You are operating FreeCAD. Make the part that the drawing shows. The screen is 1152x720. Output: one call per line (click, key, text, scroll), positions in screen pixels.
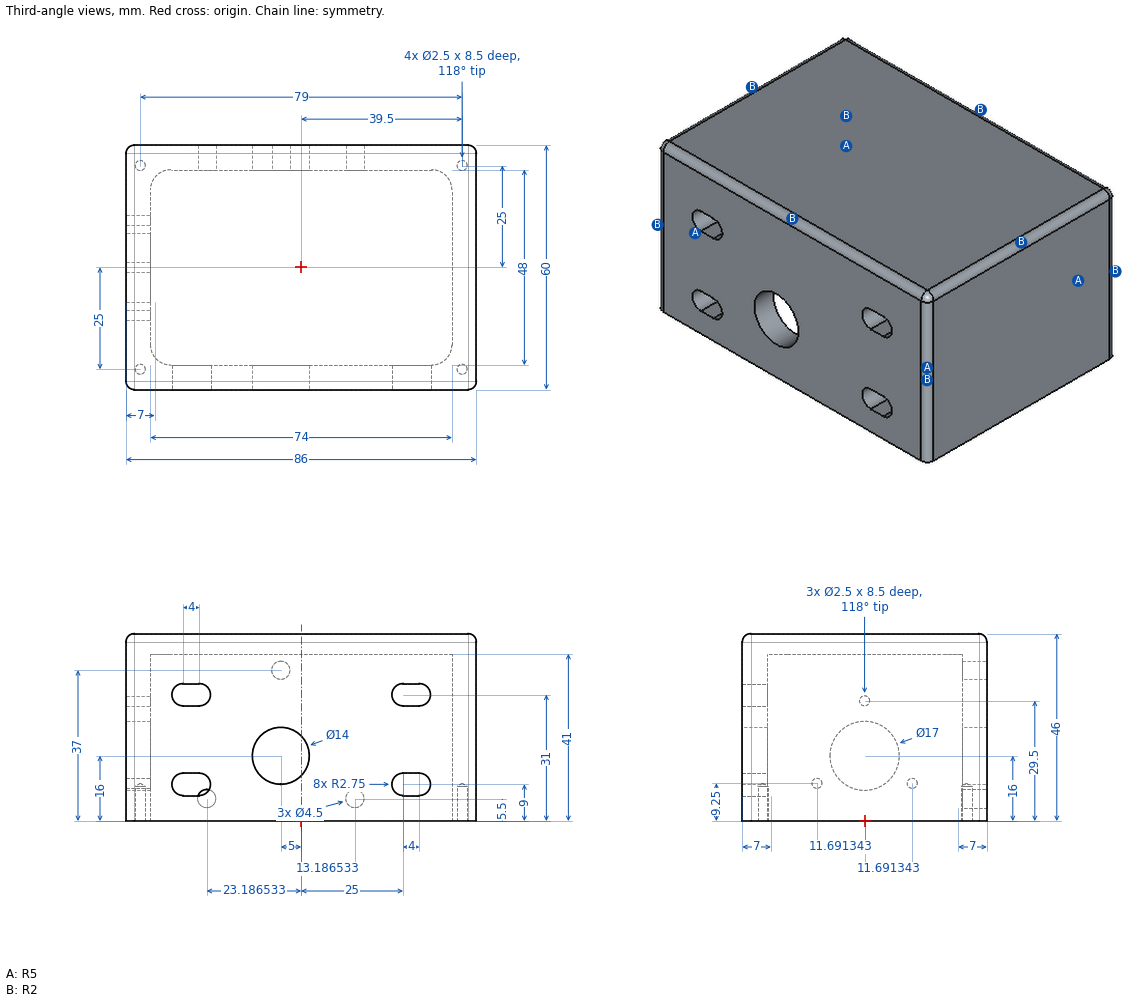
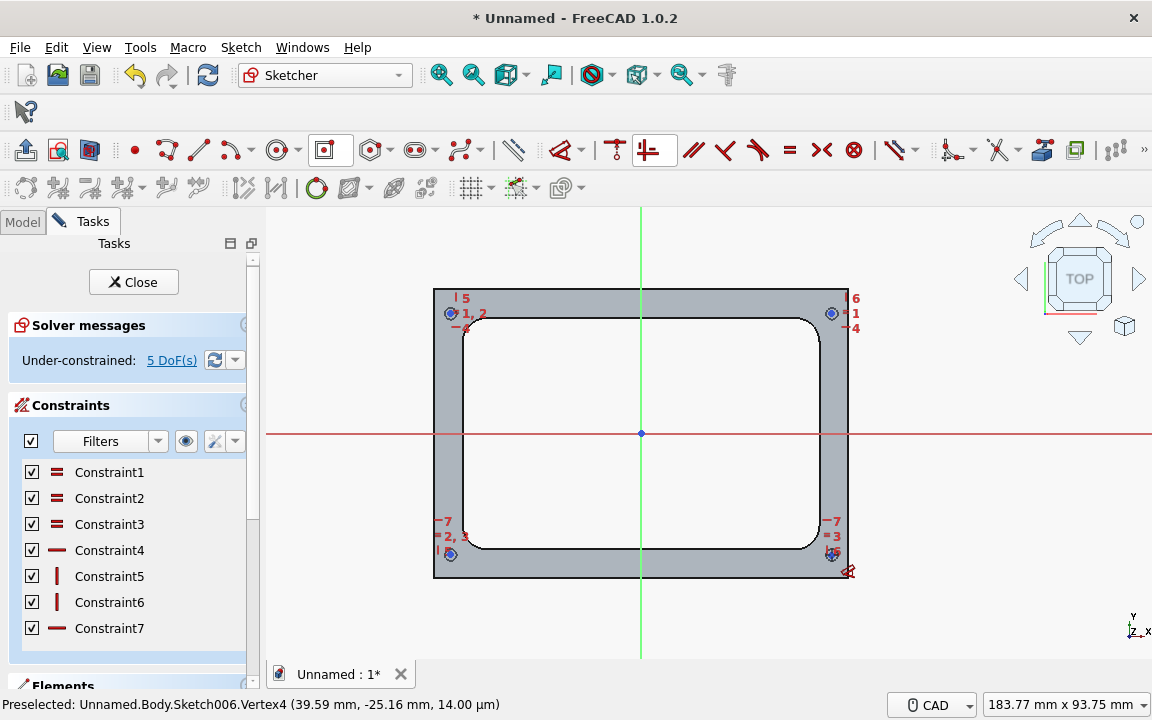
scroll(826, 314, up, 6)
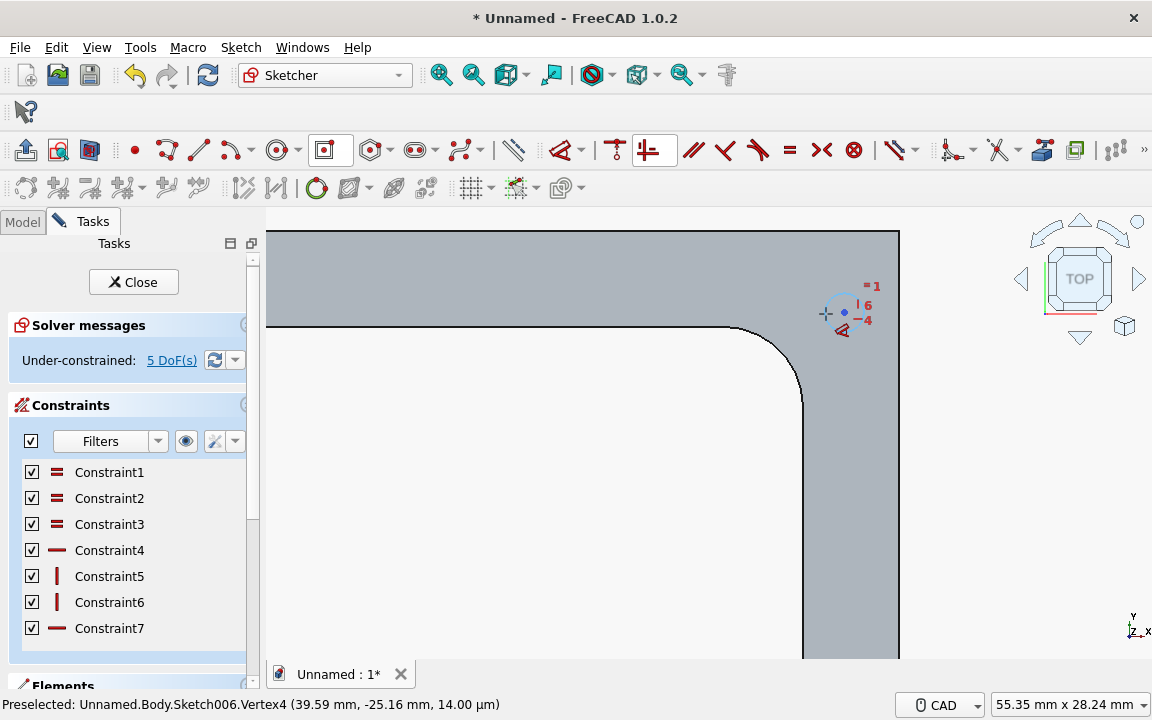
click(825, 312)
click(793, 311)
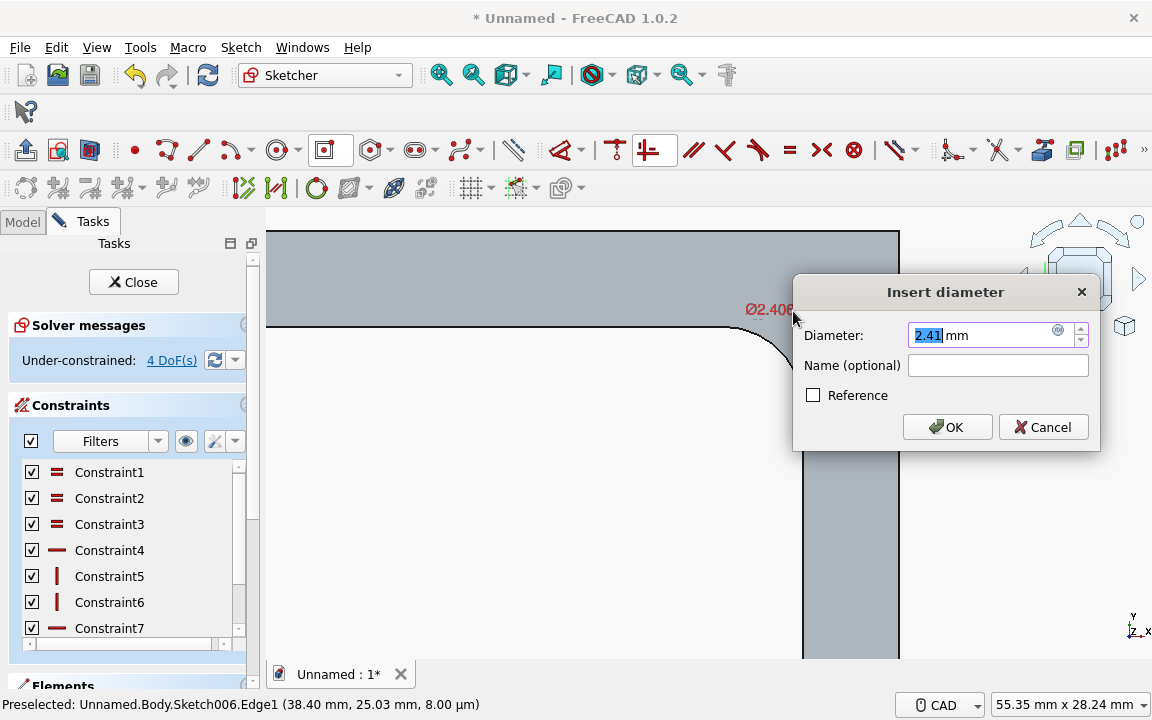
text(2.5)
key(Return)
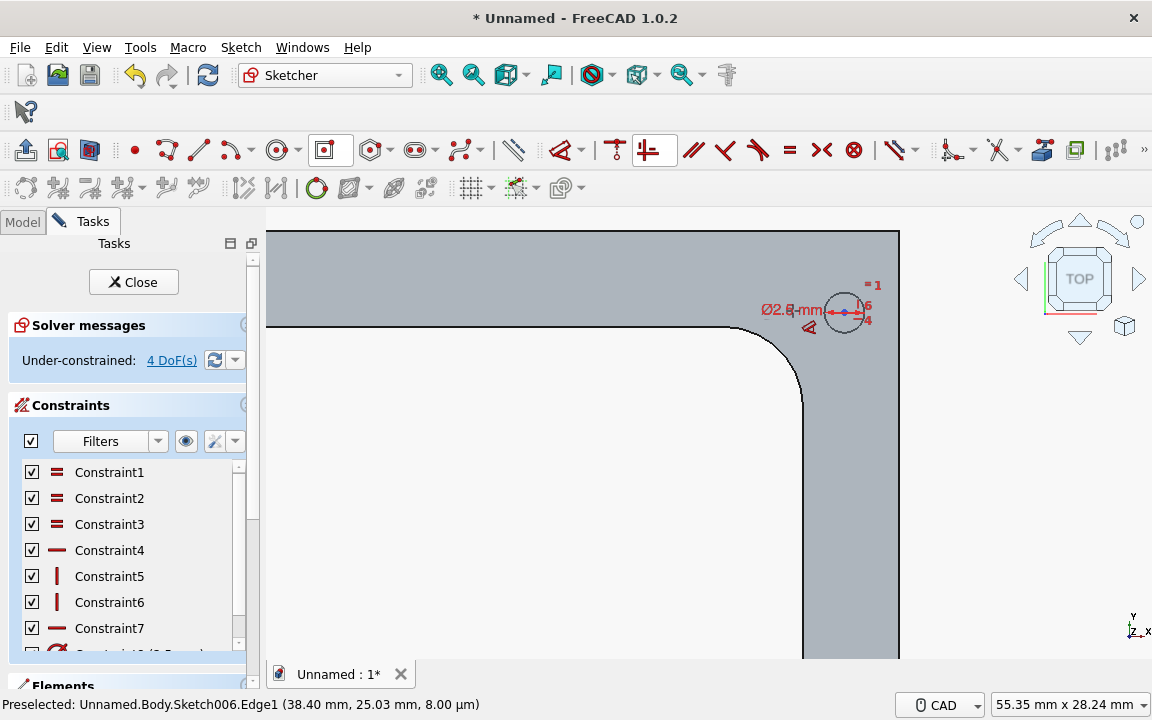
scroll(826, 313, down, 6)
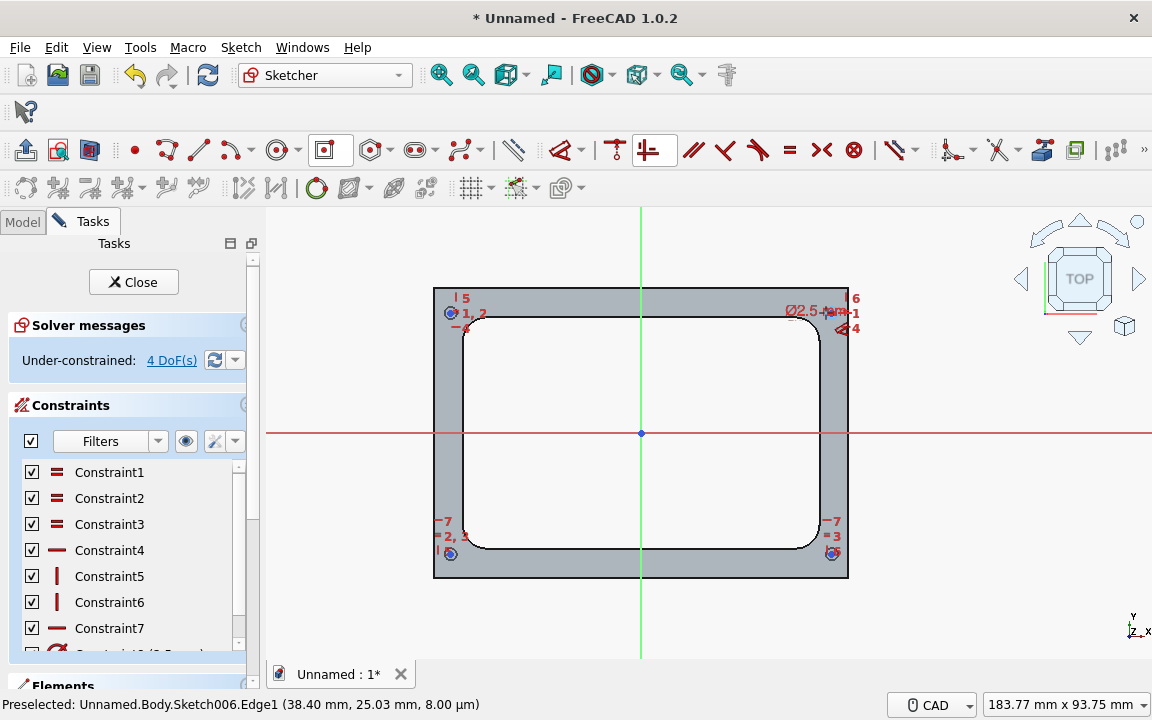
click(832, 313)
click(866, 373)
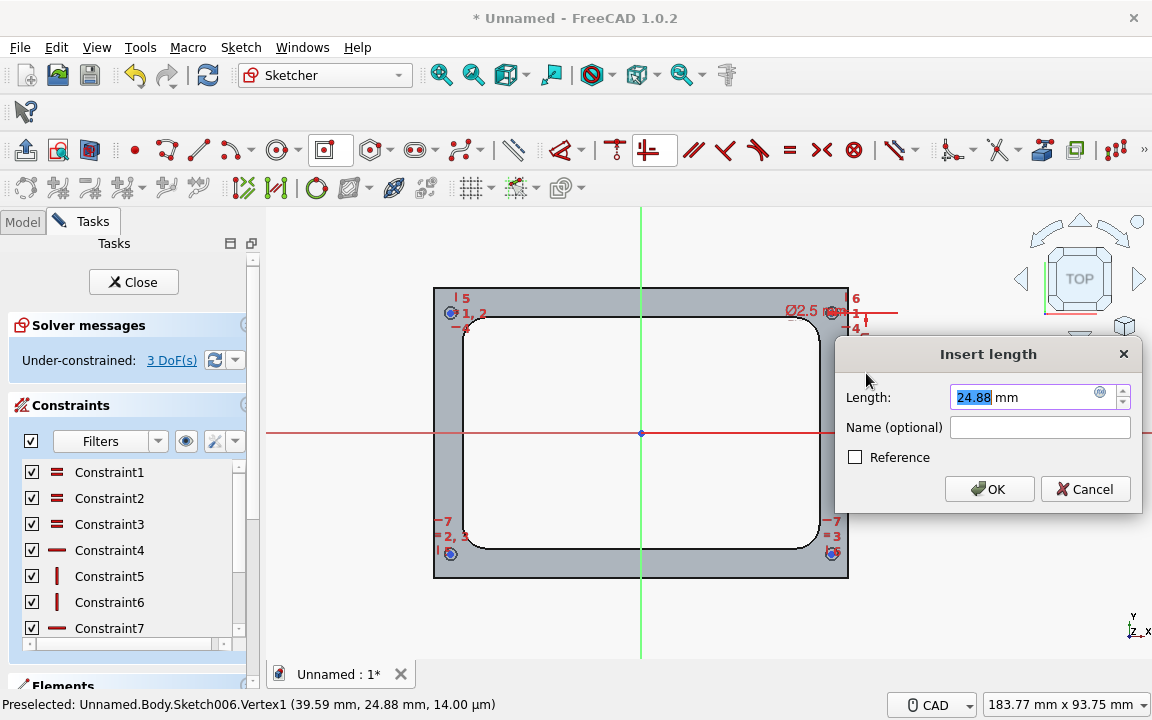
text(25)
key(Return)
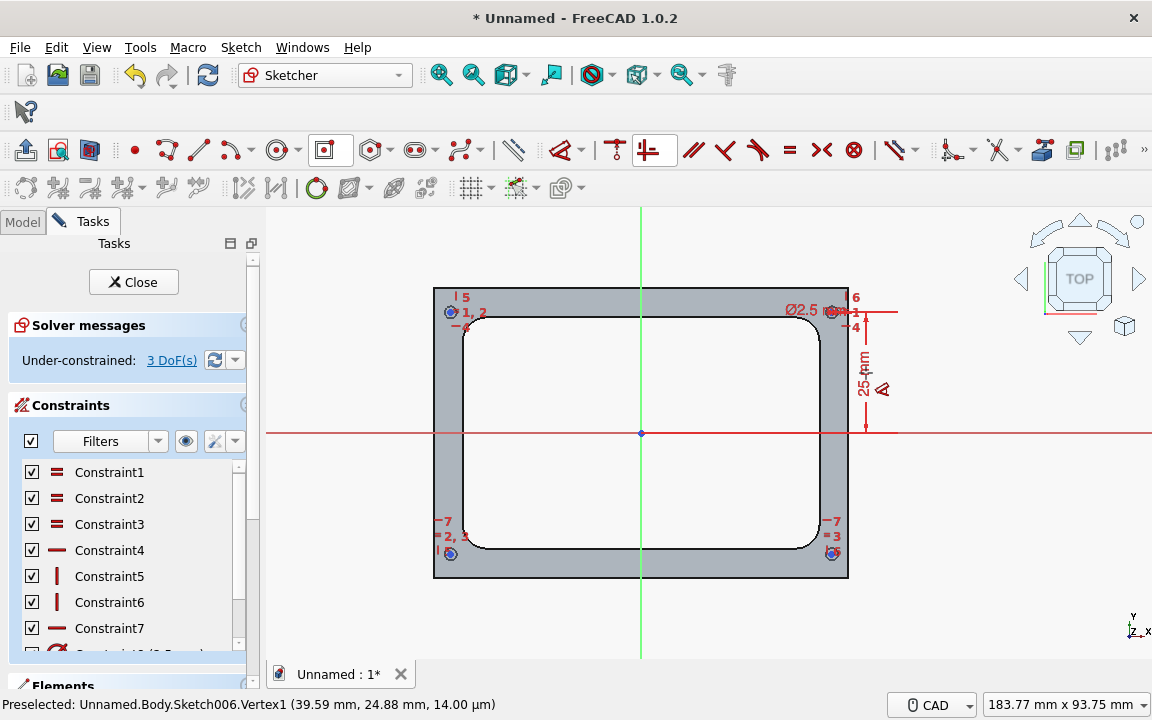
click(451, 554)
click(417, 494)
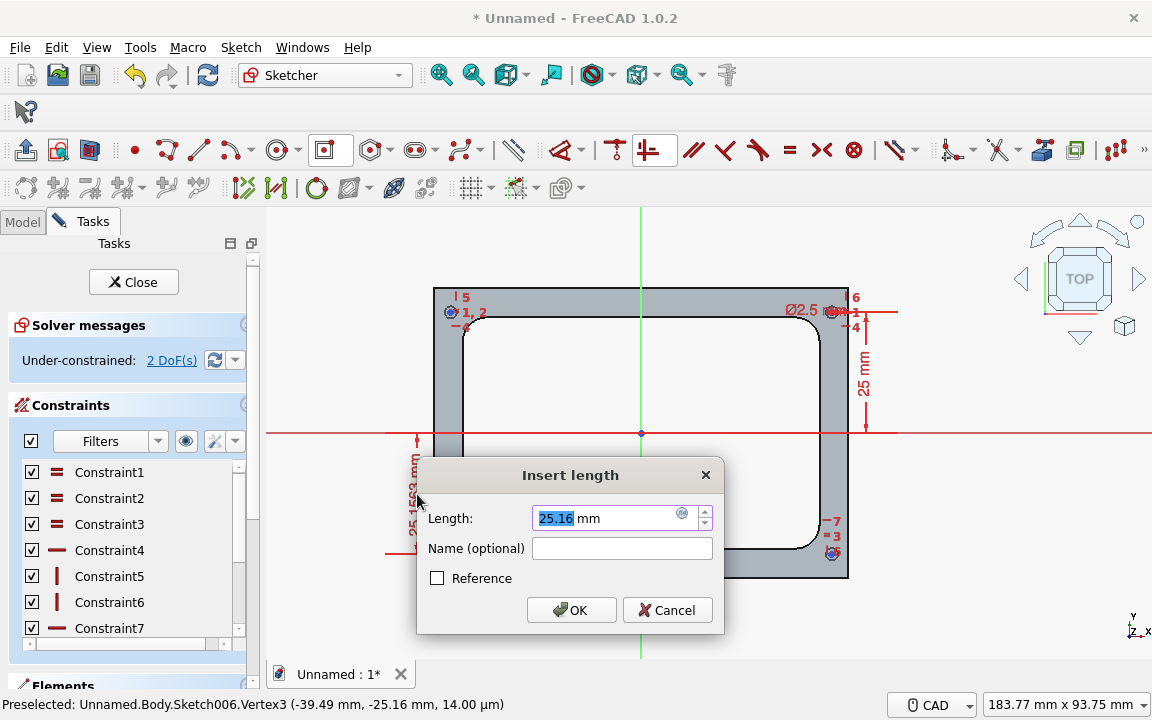
text(25)
key(Return)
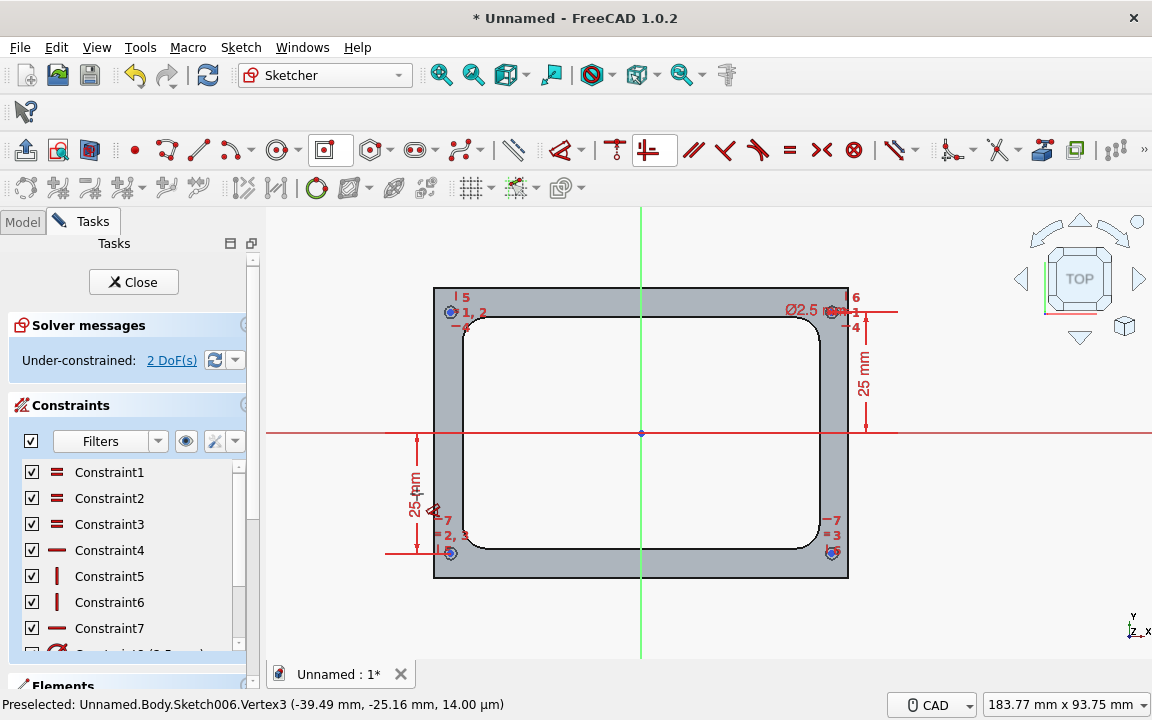
click(832, 312)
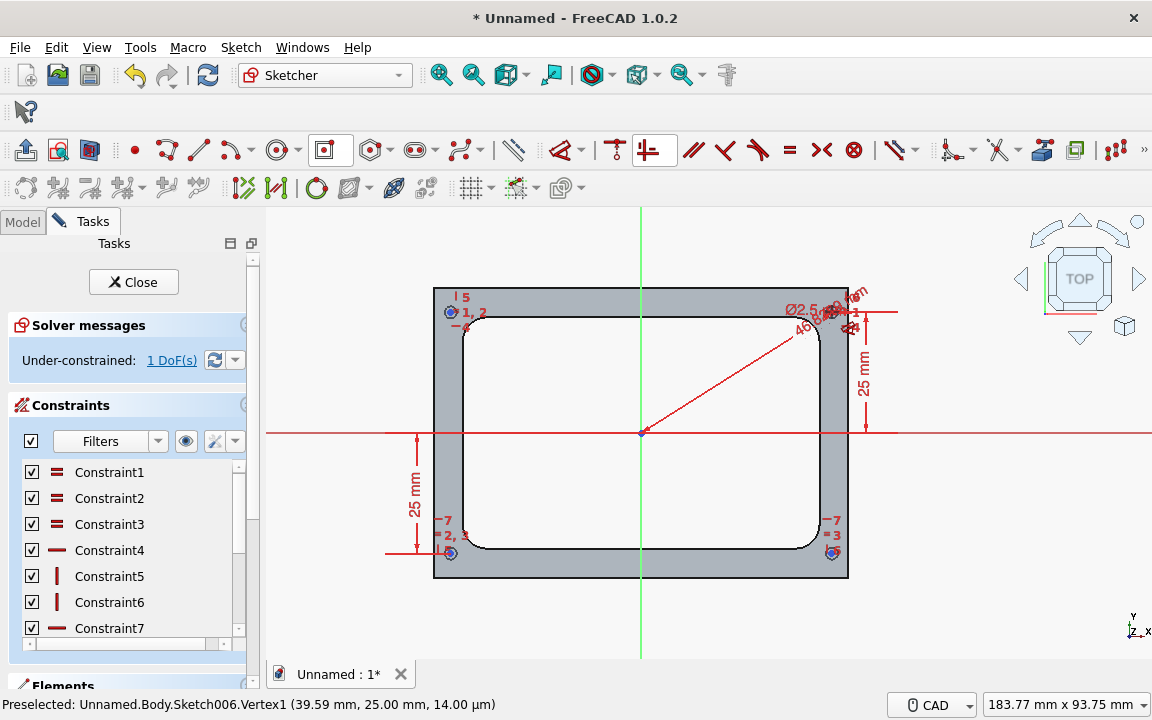
click(451, 312)
click(554, 278)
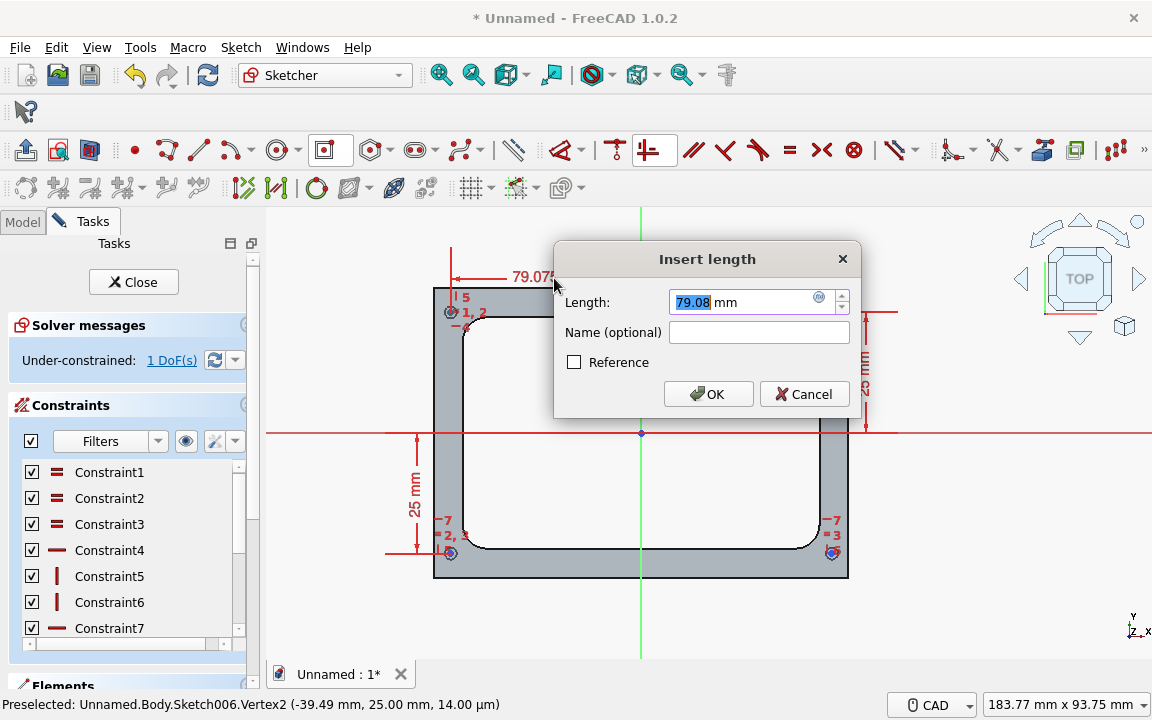
text(79)
key(Return)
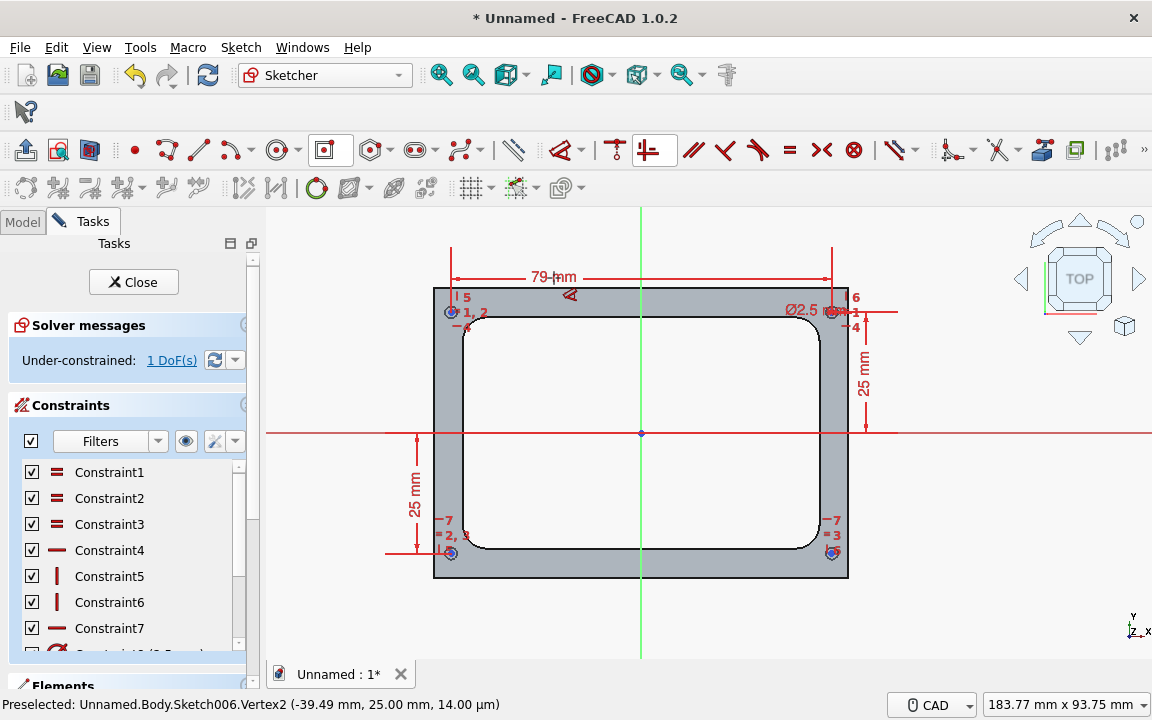
click(832, 312)
click(737, 278)